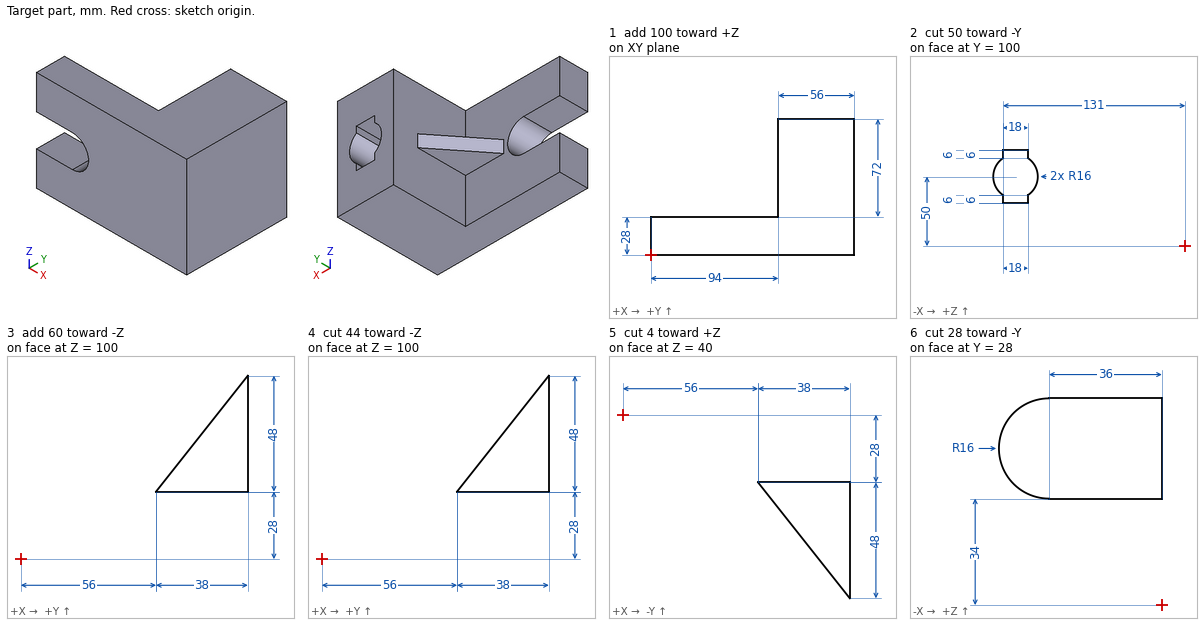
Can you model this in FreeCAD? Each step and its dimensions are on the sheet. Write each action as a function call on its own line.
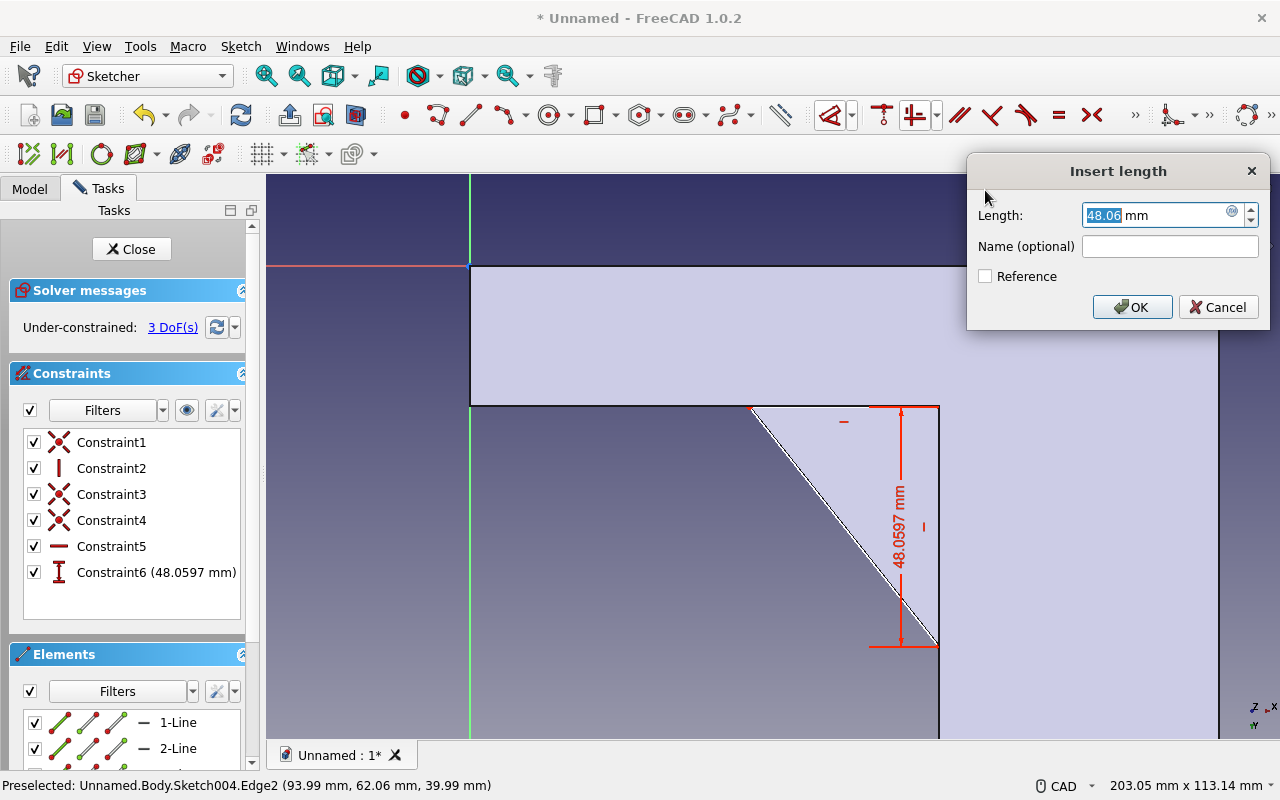
text(48)
key(Return)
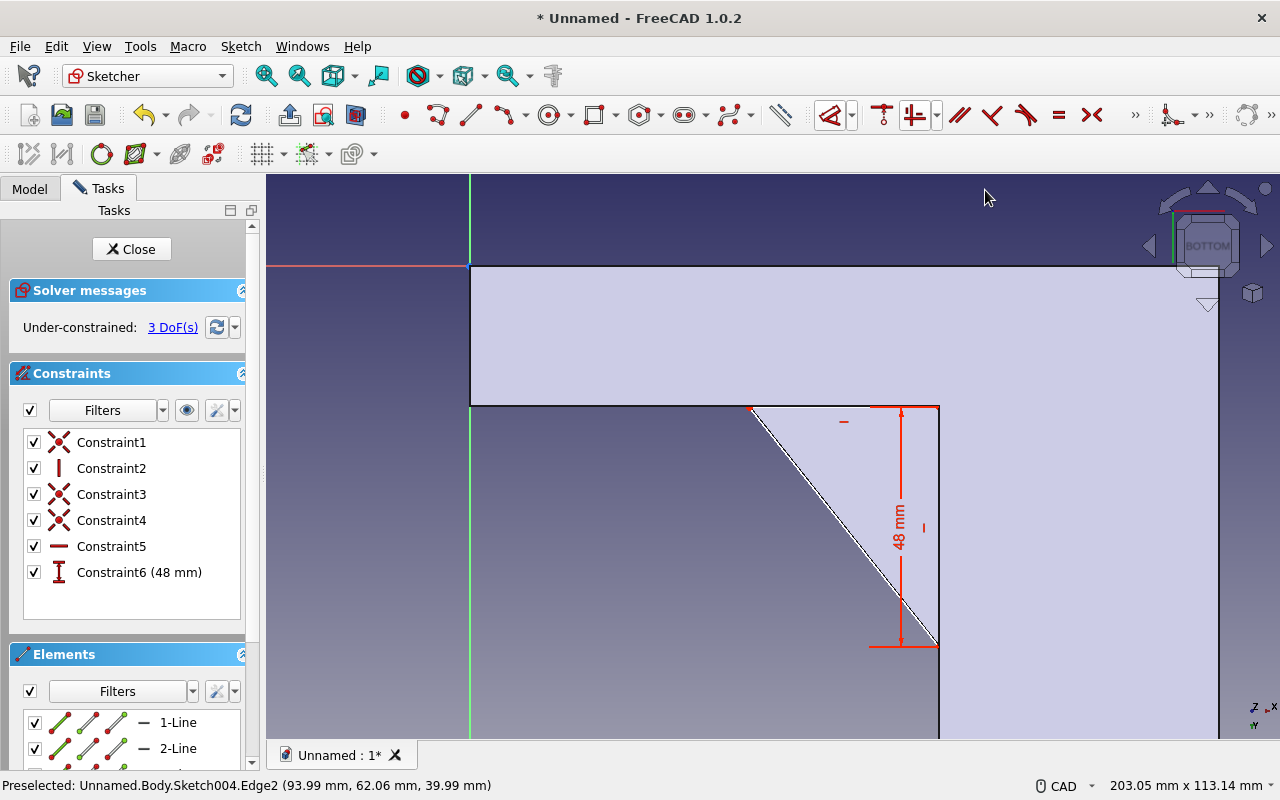
click(882, 407)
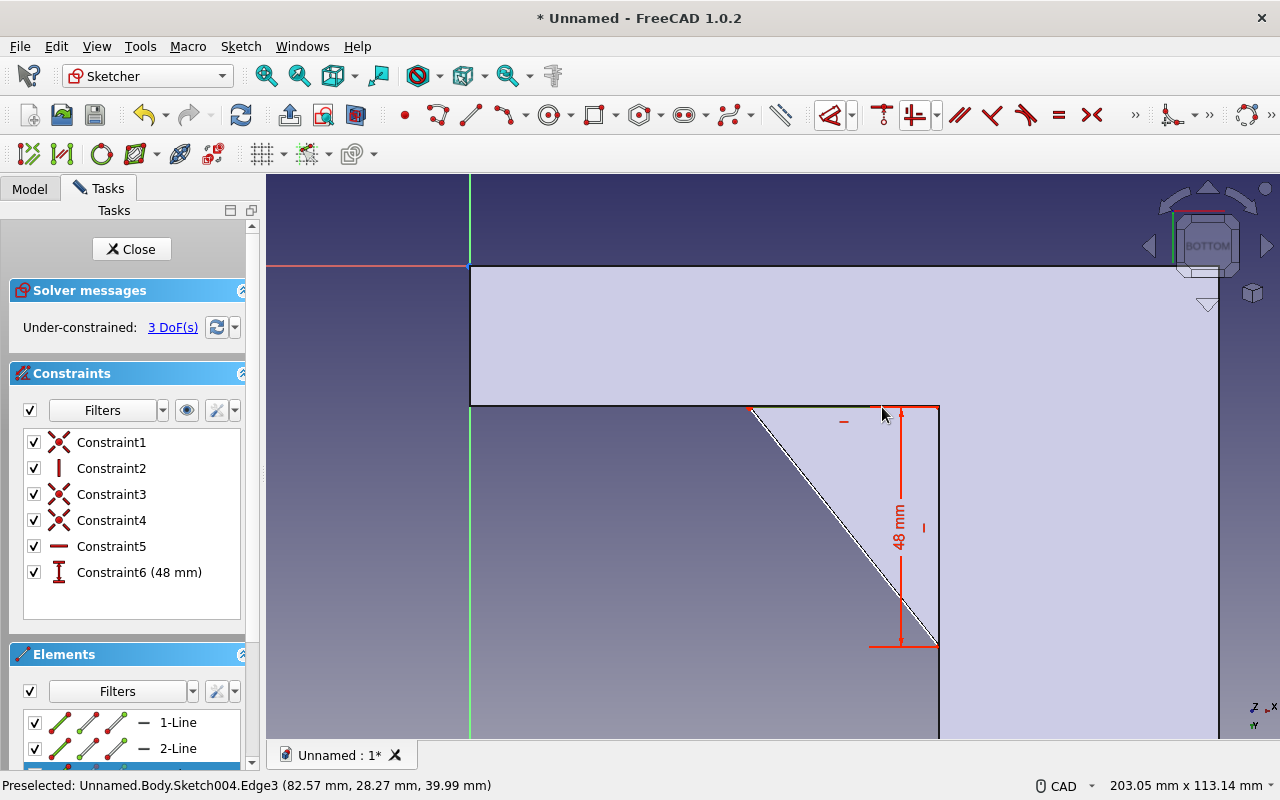
click(852, 116)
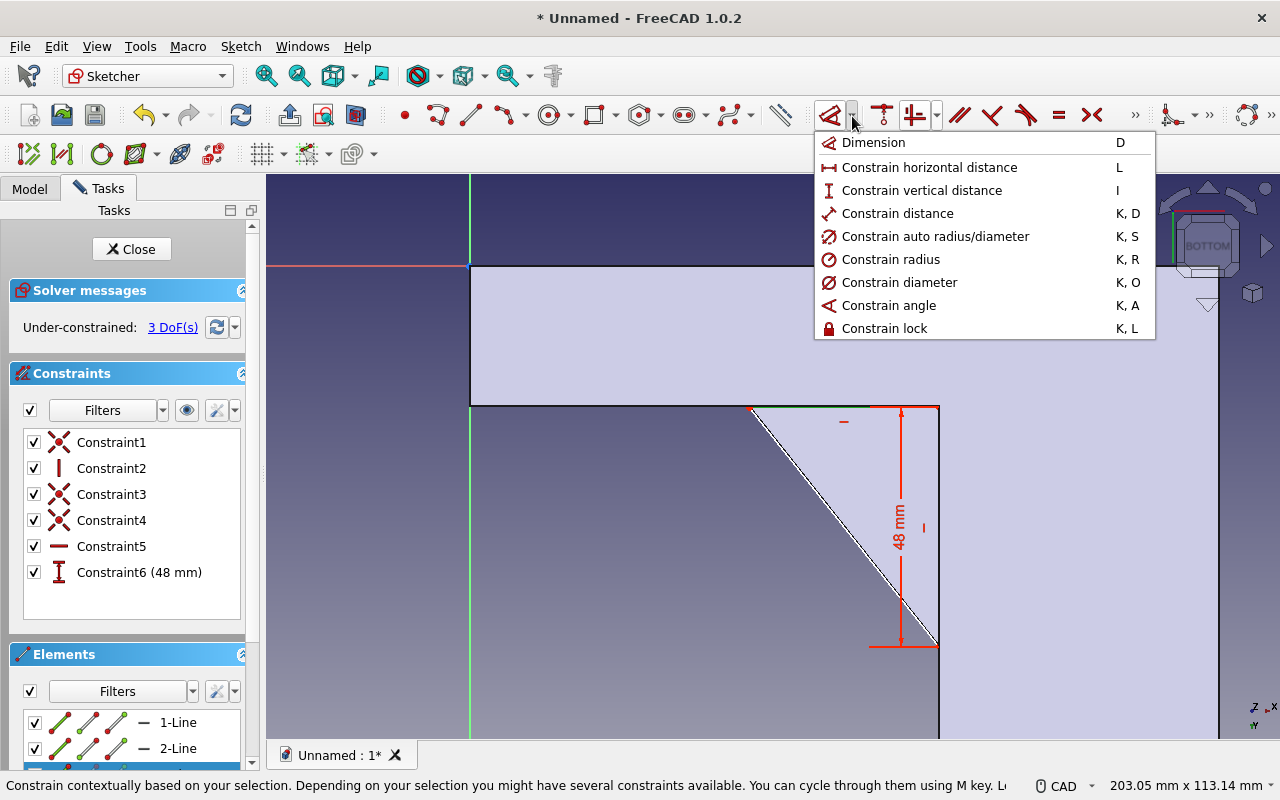
click(985, 168)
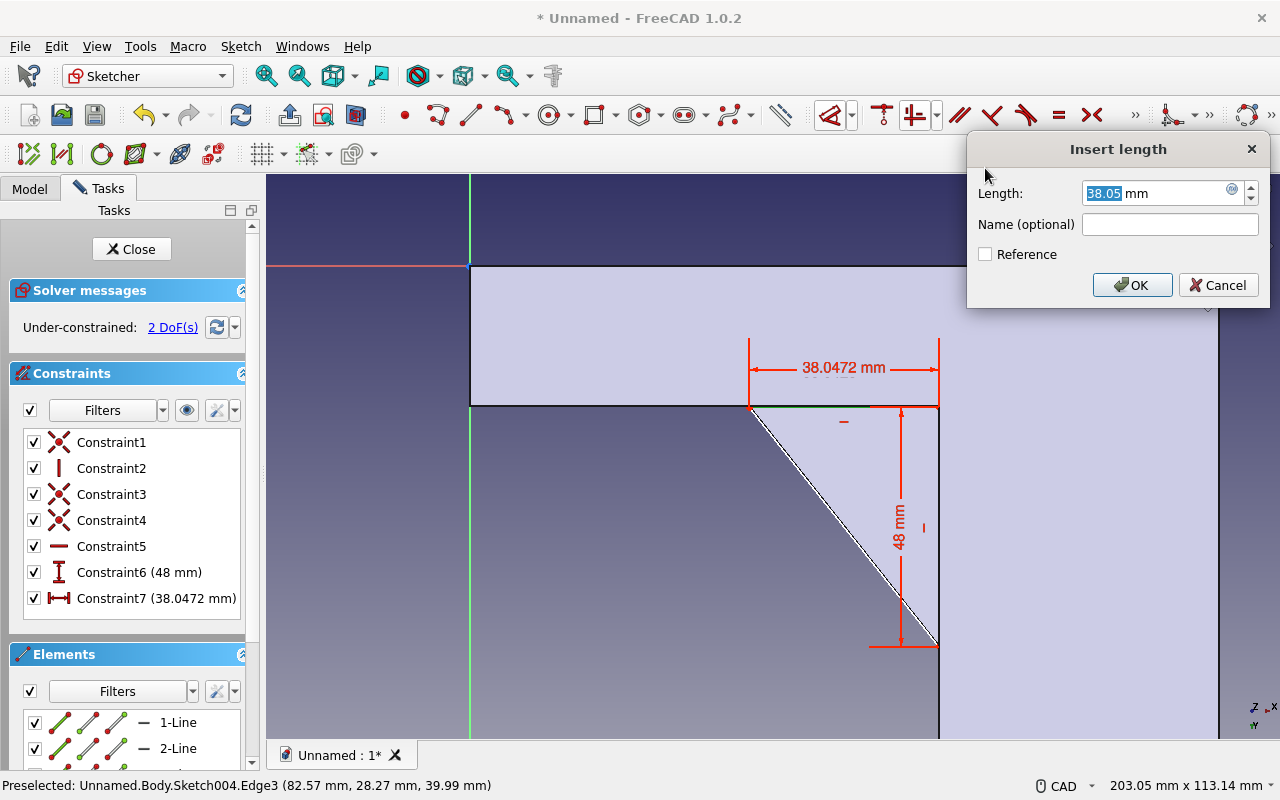
text(38)
key(Return)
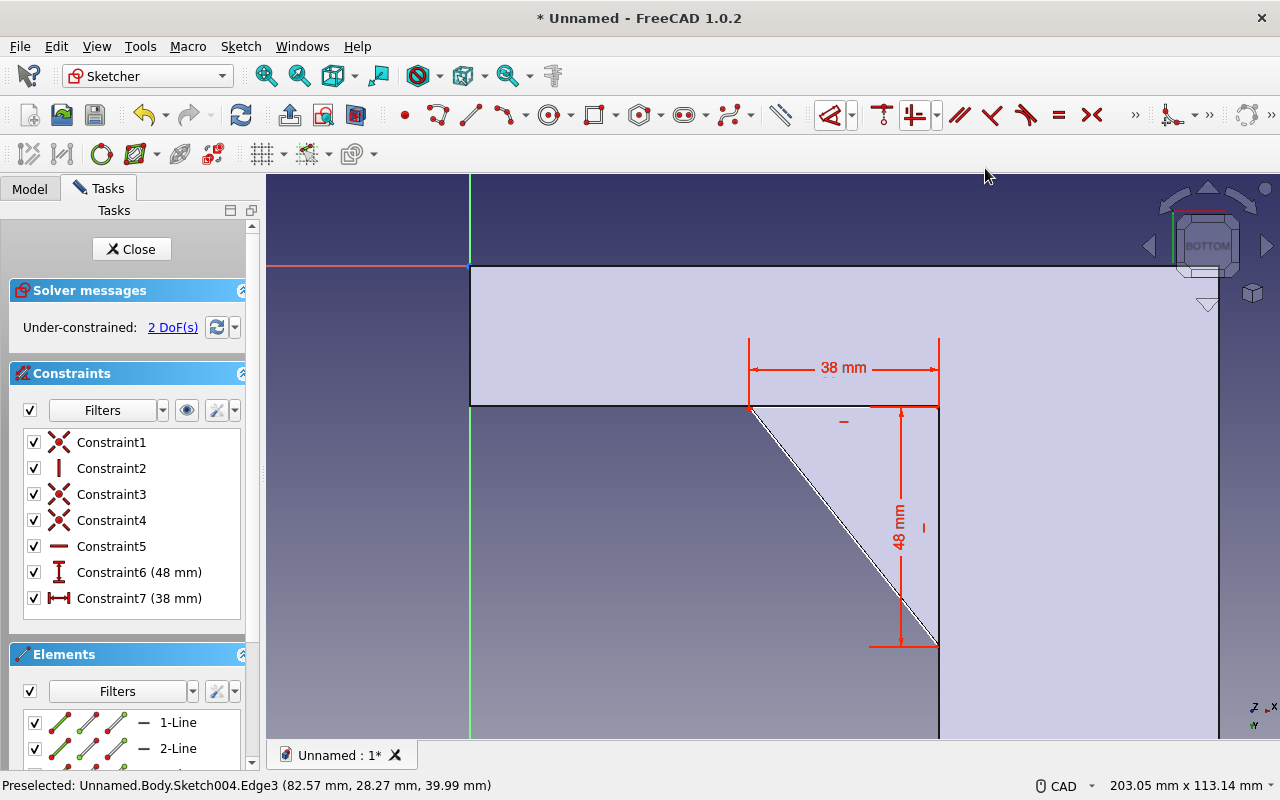
click(749, 407)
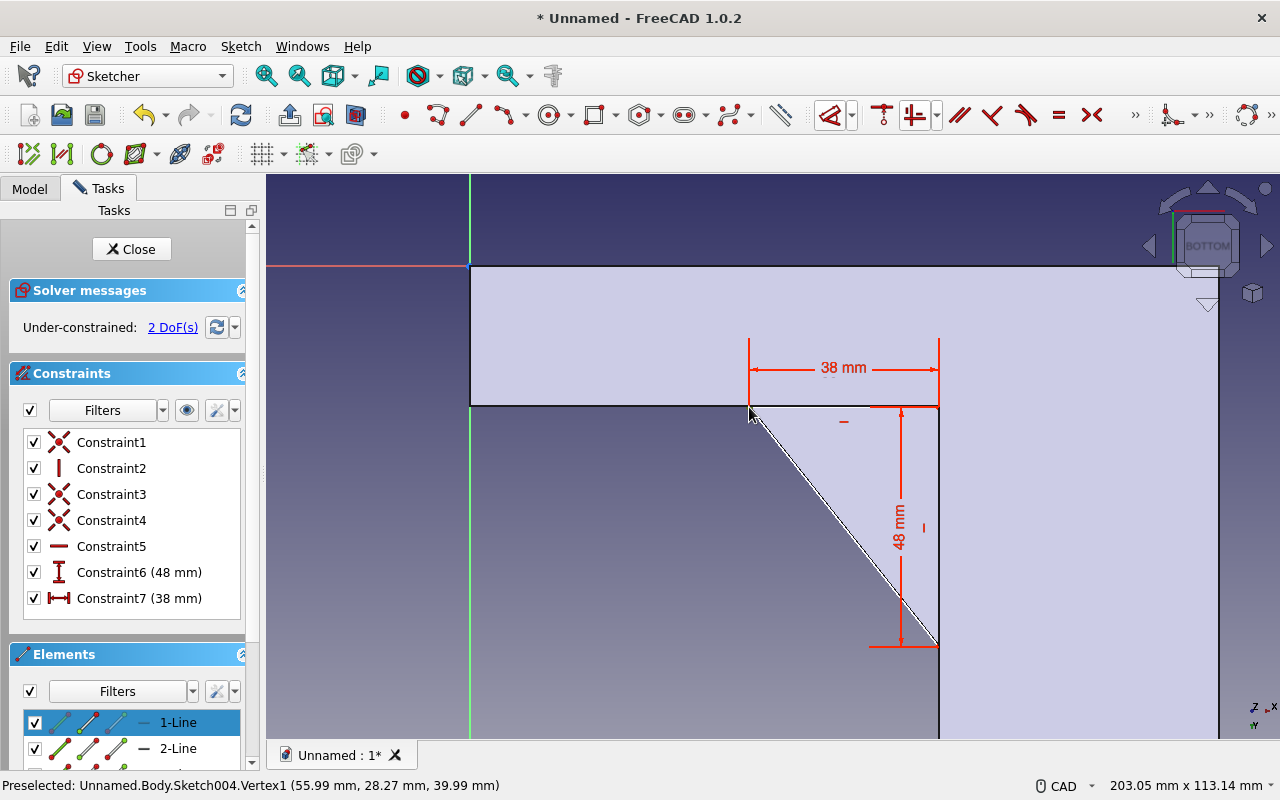
click(852, 116)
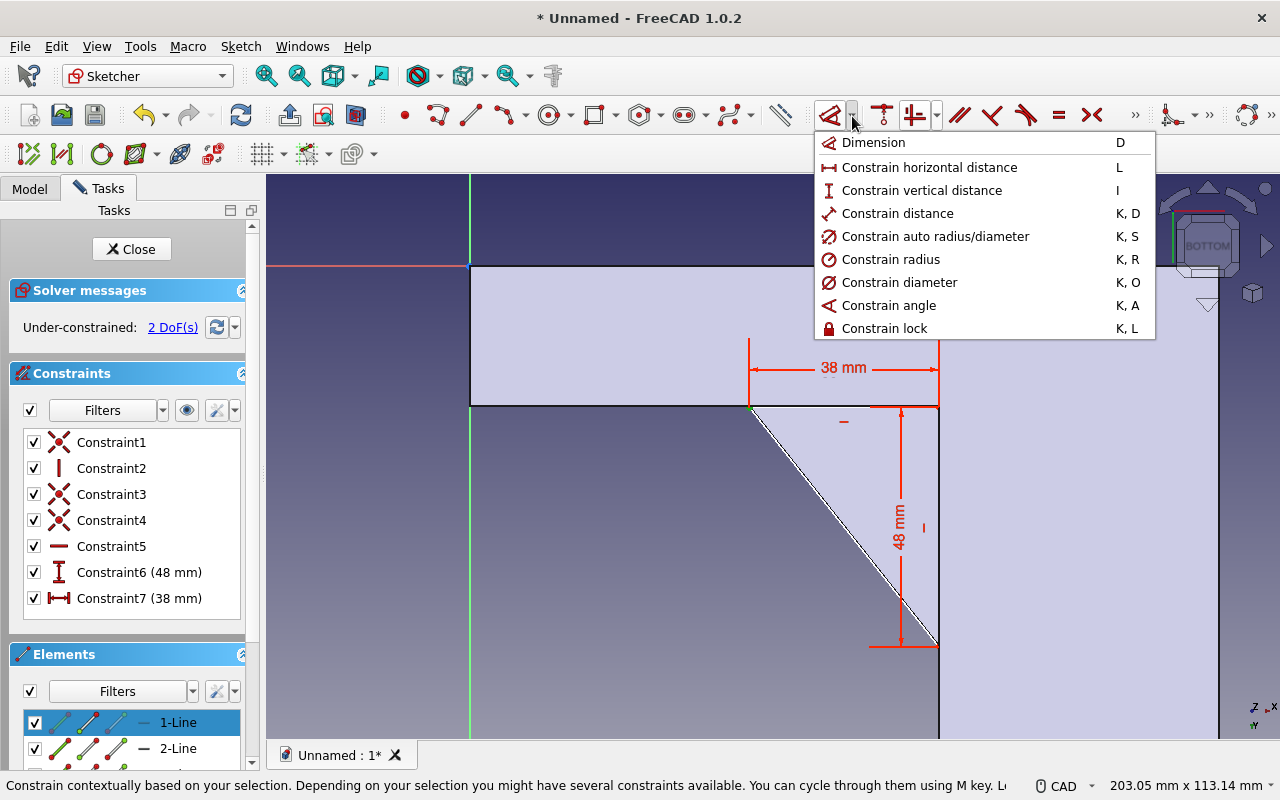
click(985, 168)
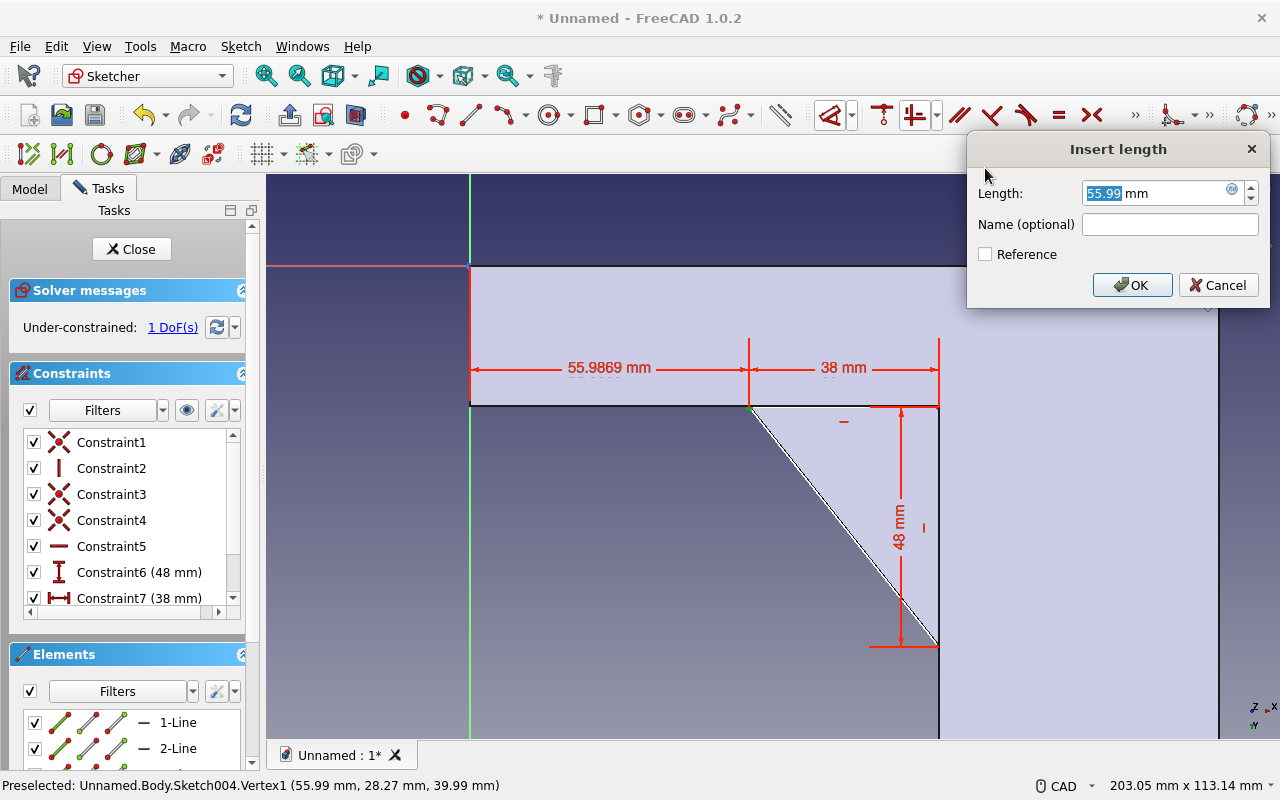
text(56)
key(Return)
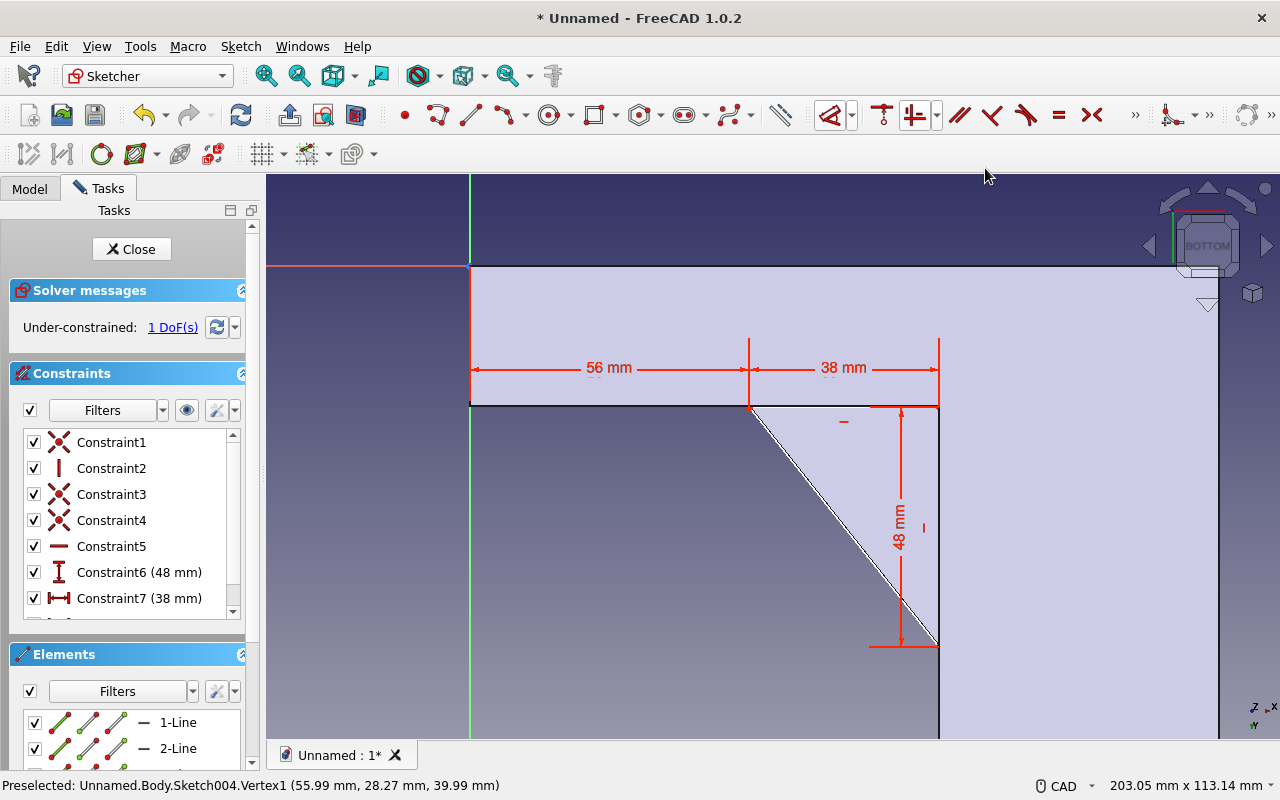
click(749, 407)